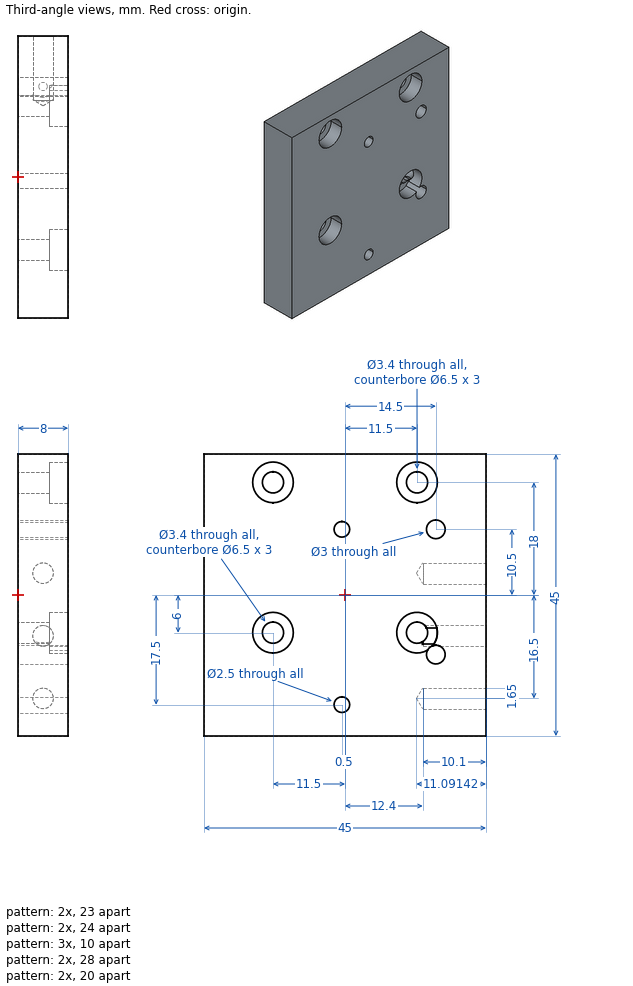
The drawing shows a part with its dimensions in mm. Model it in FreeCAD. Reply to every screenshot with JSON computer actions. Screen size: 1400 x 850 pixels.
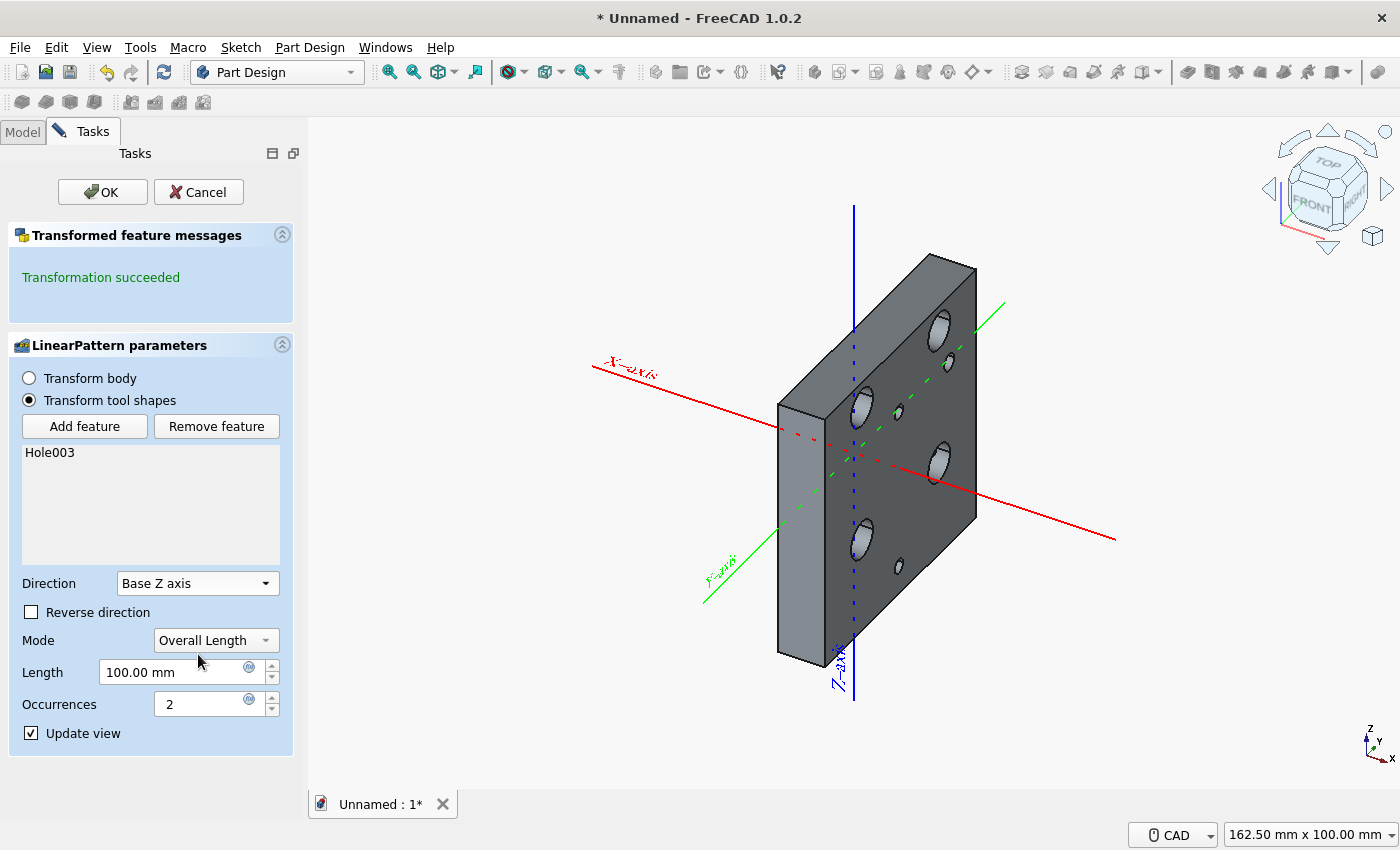
{"action": "left_click", "coordinate": [217, 640]}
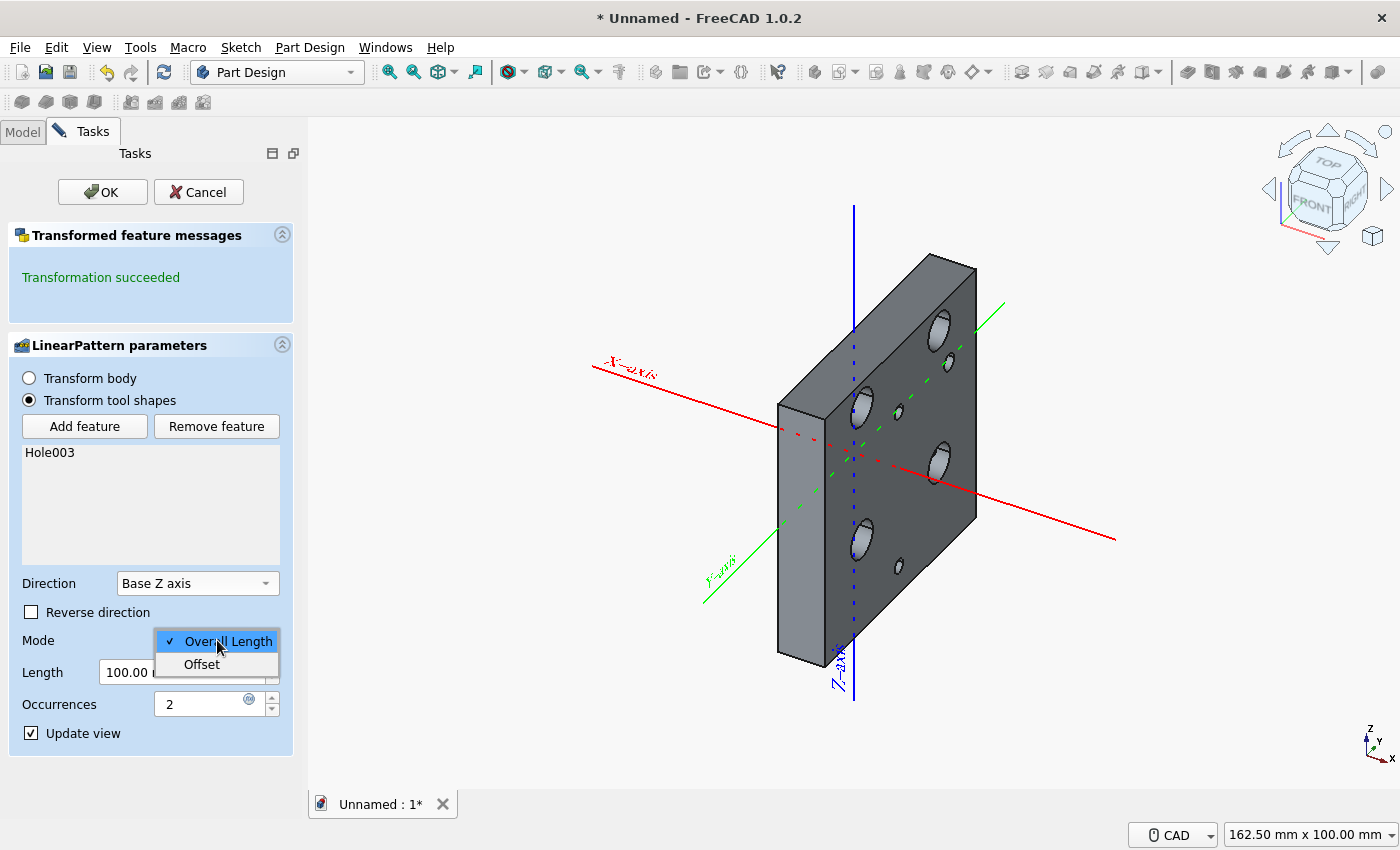
{"action": "left_click", "coordinate": [216, 664]}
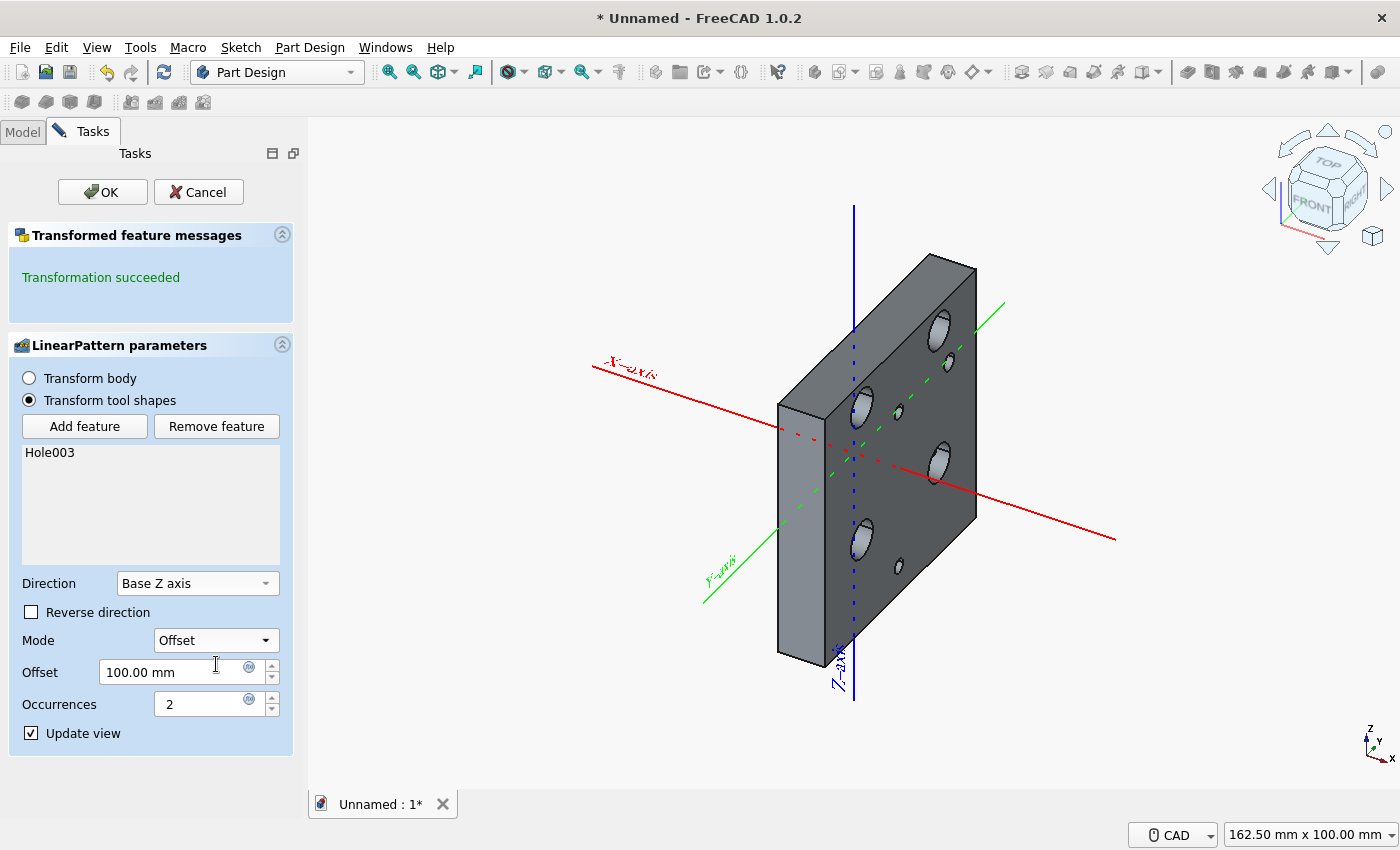
{"action": "triple_click", "coordinate": [182, 672]}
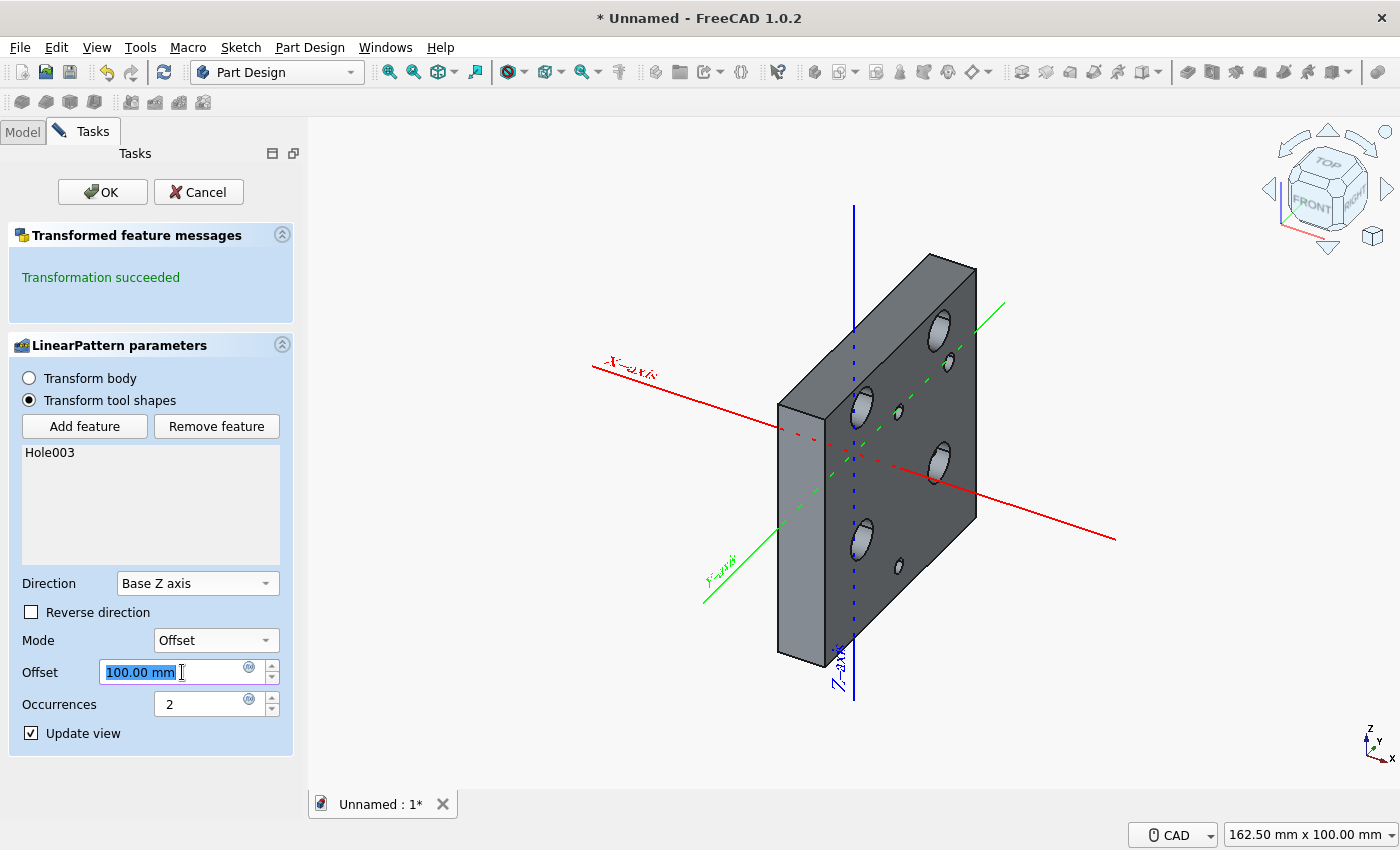
{"action": "type", "text": "20"}
{"action": "key", "text": "Tab"}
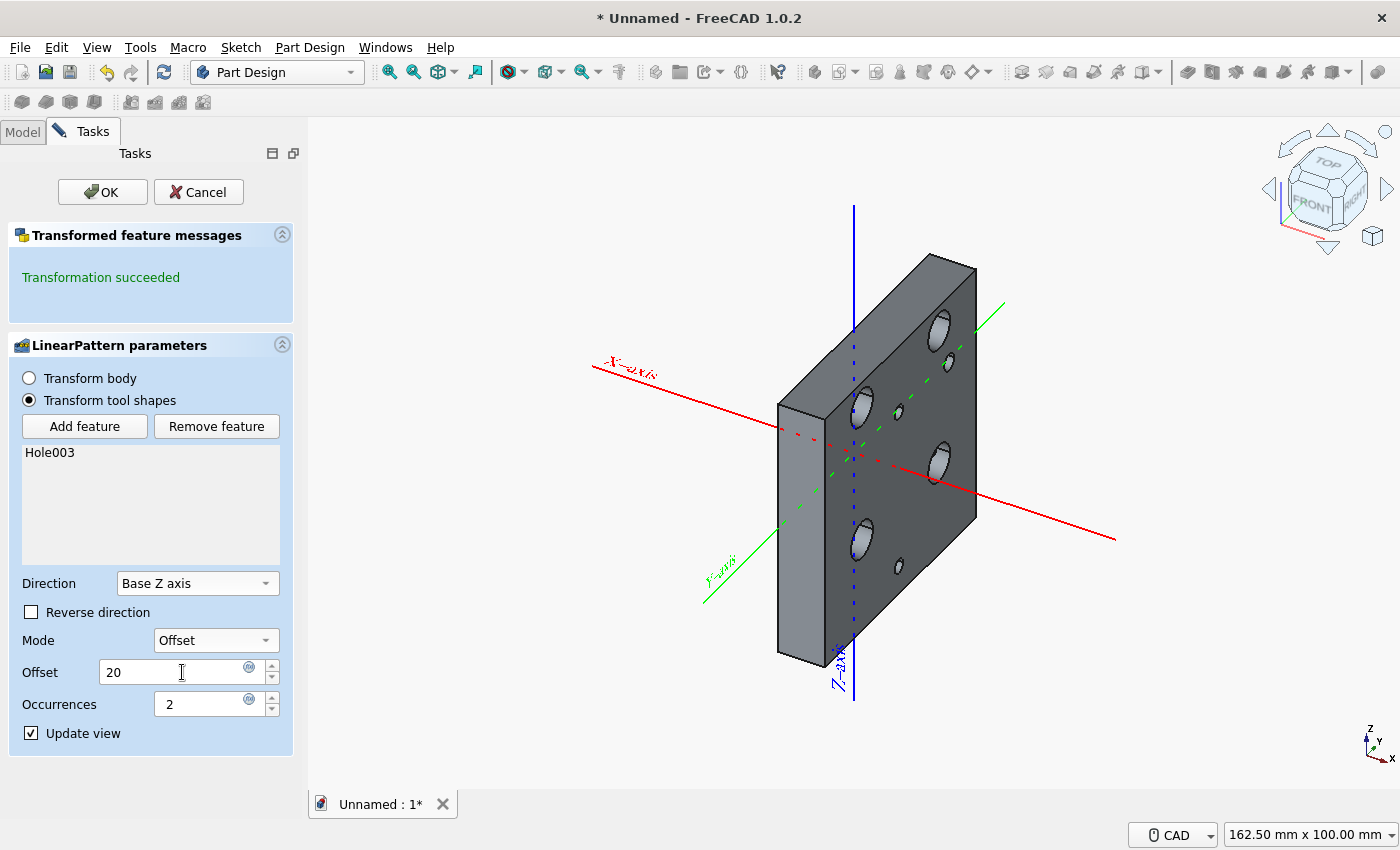
{"action": "triple_click", "coordinate": [209, 704]}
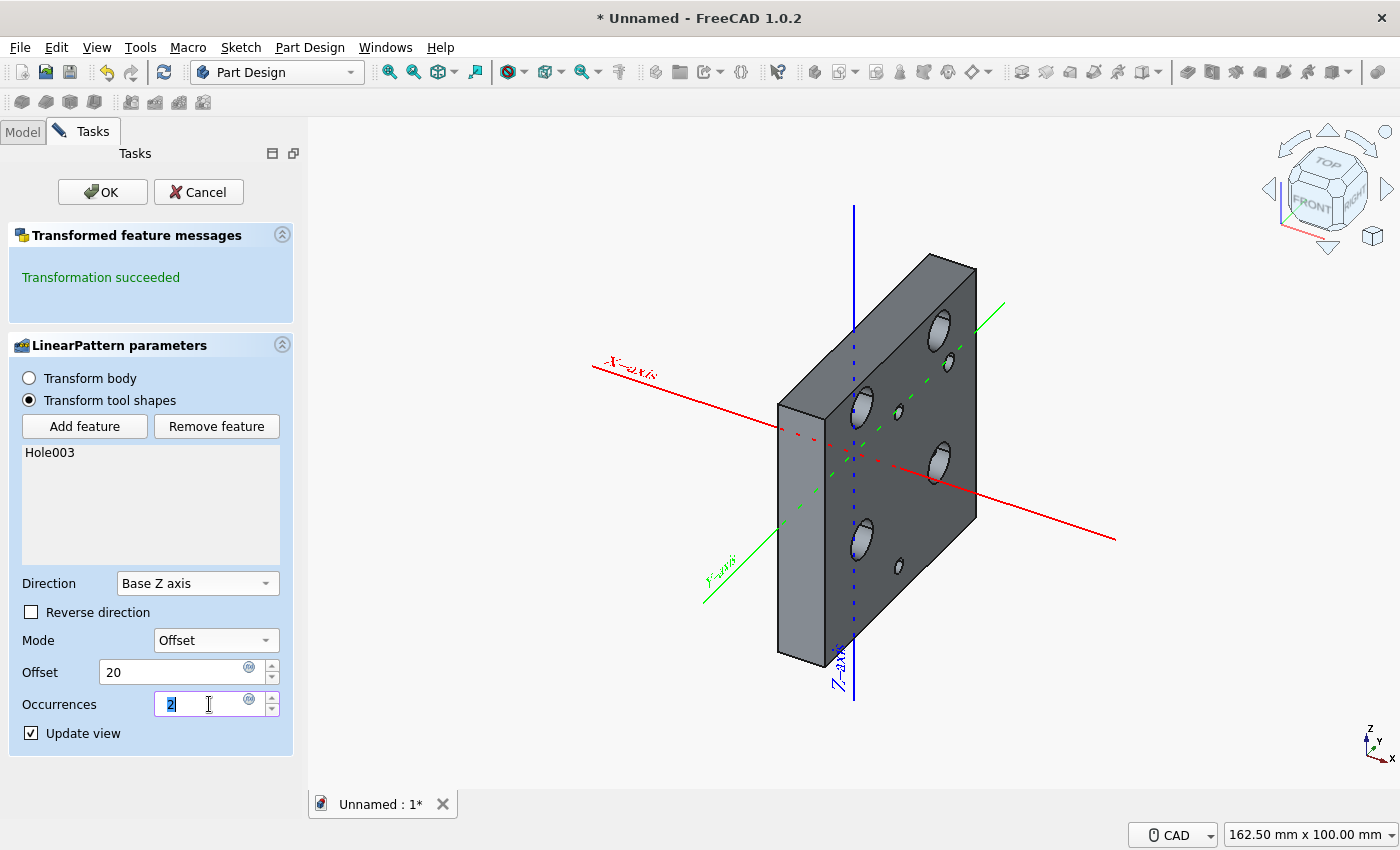
{"action": "type", "text": "2"}
{"action": "key", "text": "Tab"}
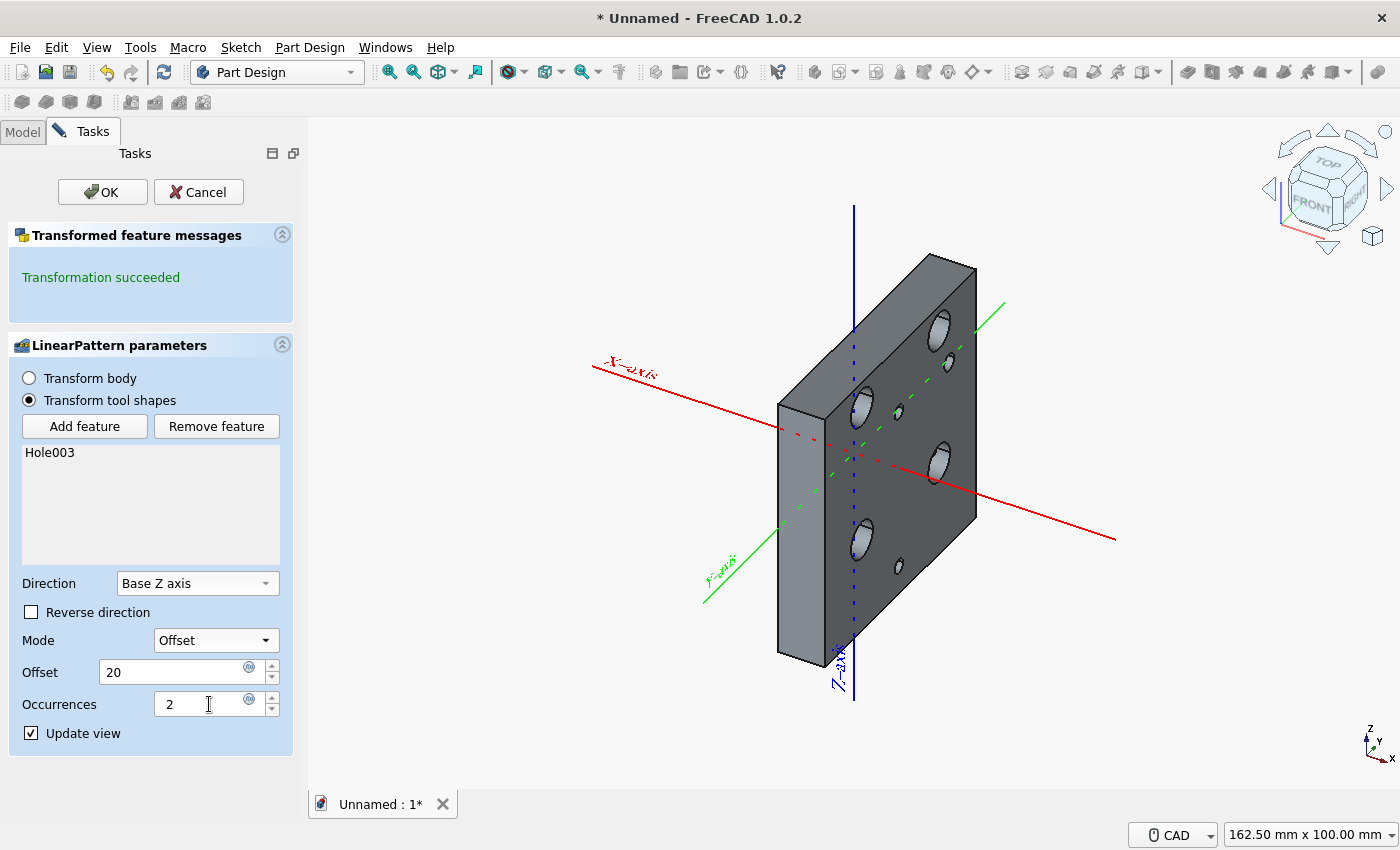
{"action": "left_click", "coordinate": [30, 612]}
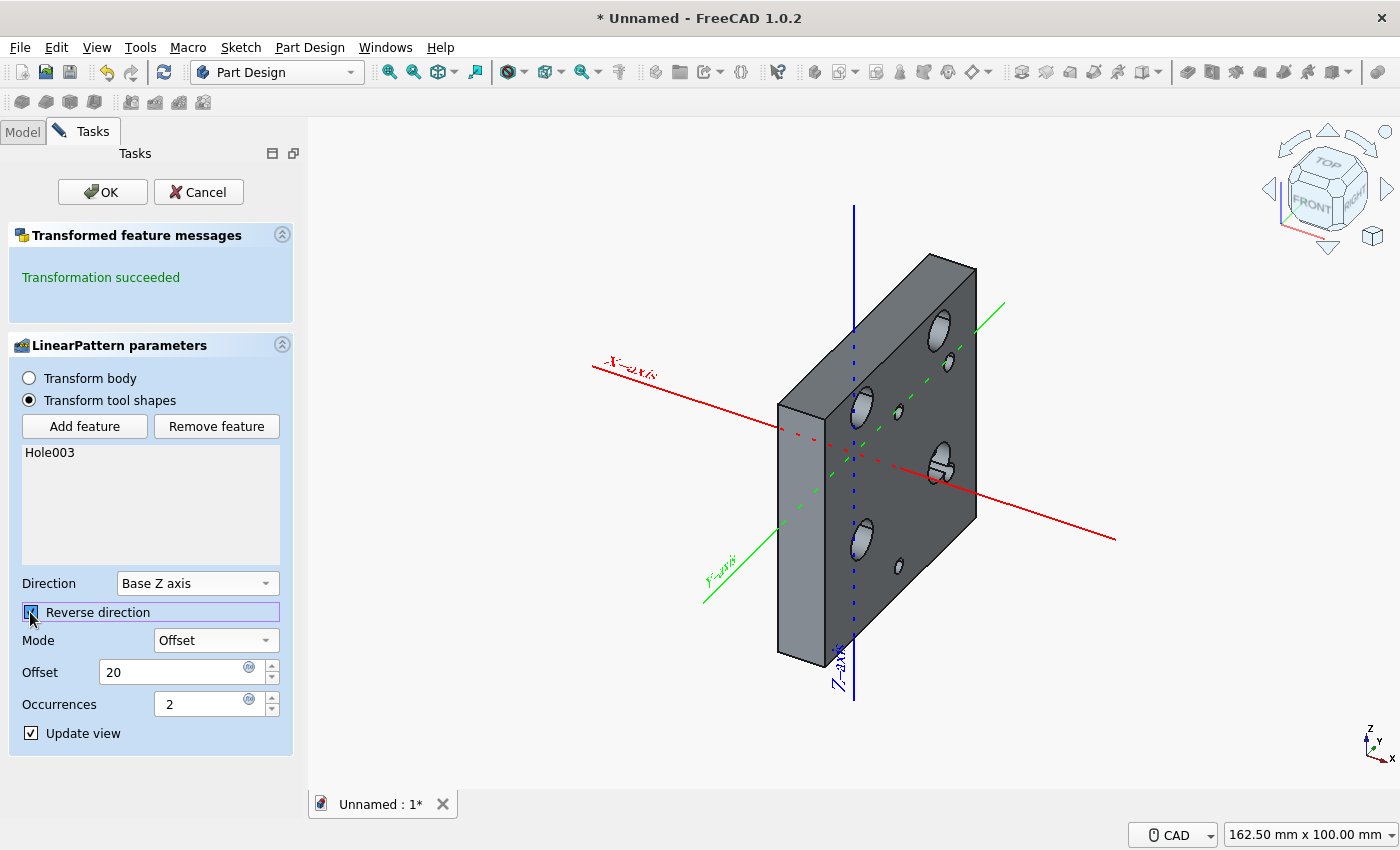
{"action": "left_click", "coordinate": [103, 192]}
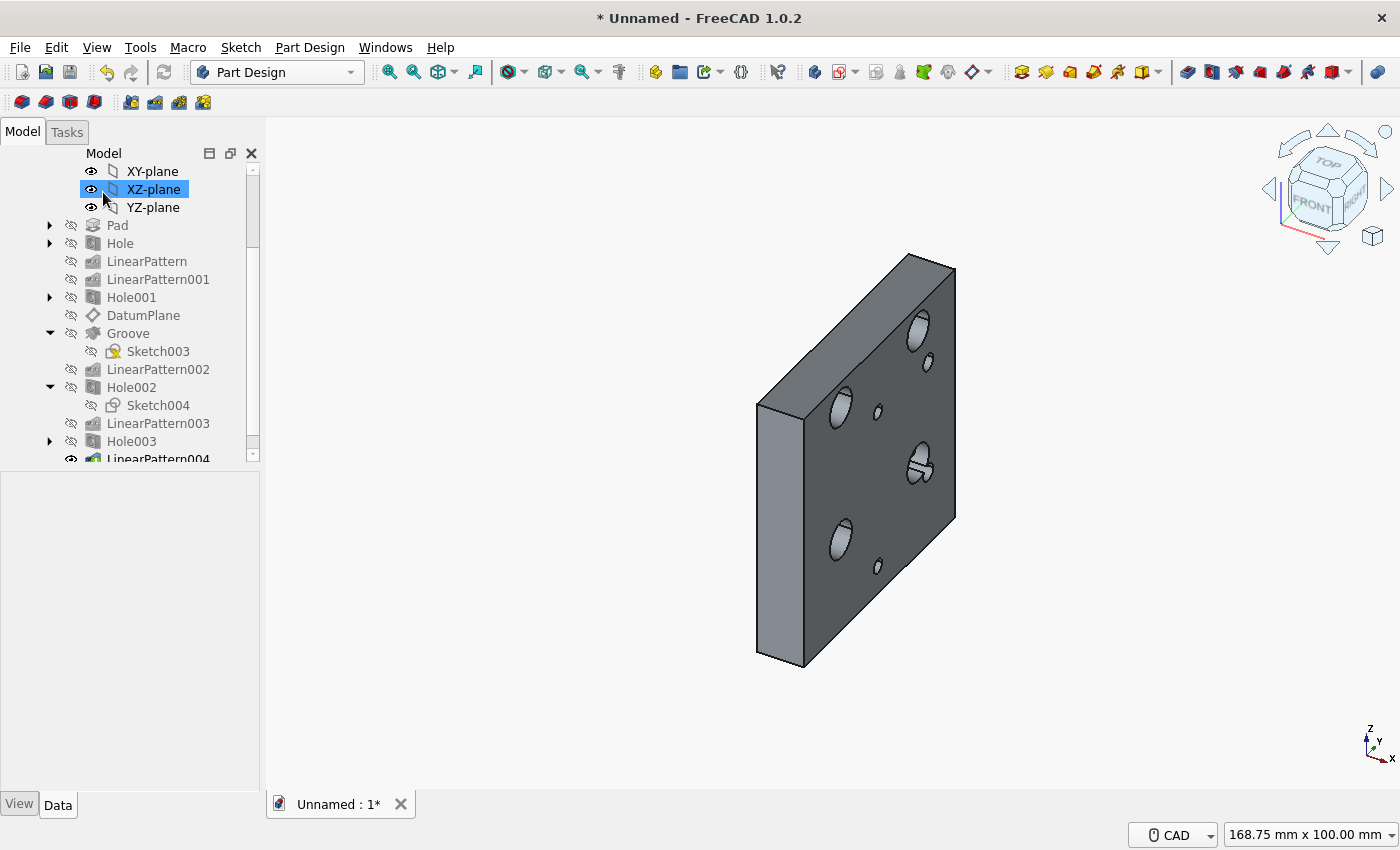
{"action": "key", "text": "0"}